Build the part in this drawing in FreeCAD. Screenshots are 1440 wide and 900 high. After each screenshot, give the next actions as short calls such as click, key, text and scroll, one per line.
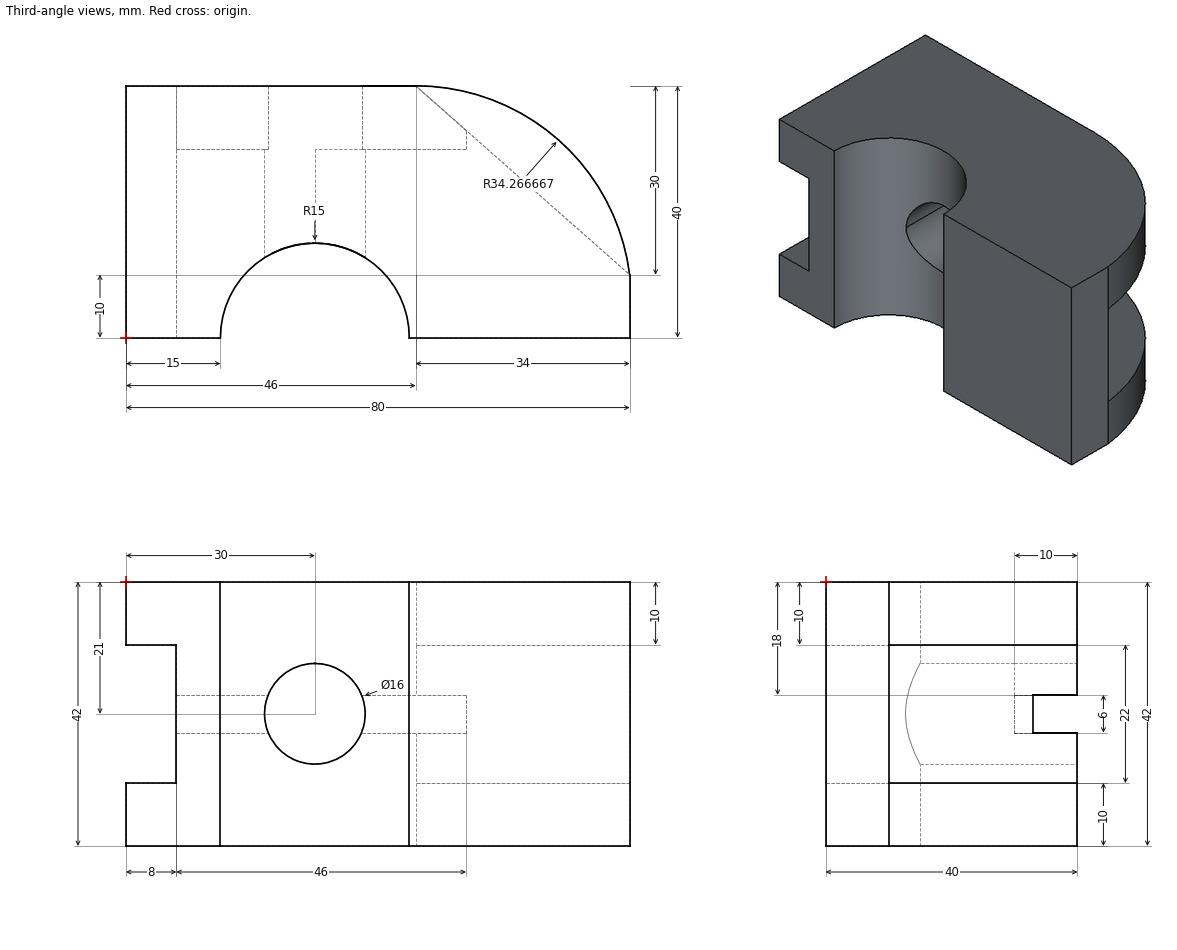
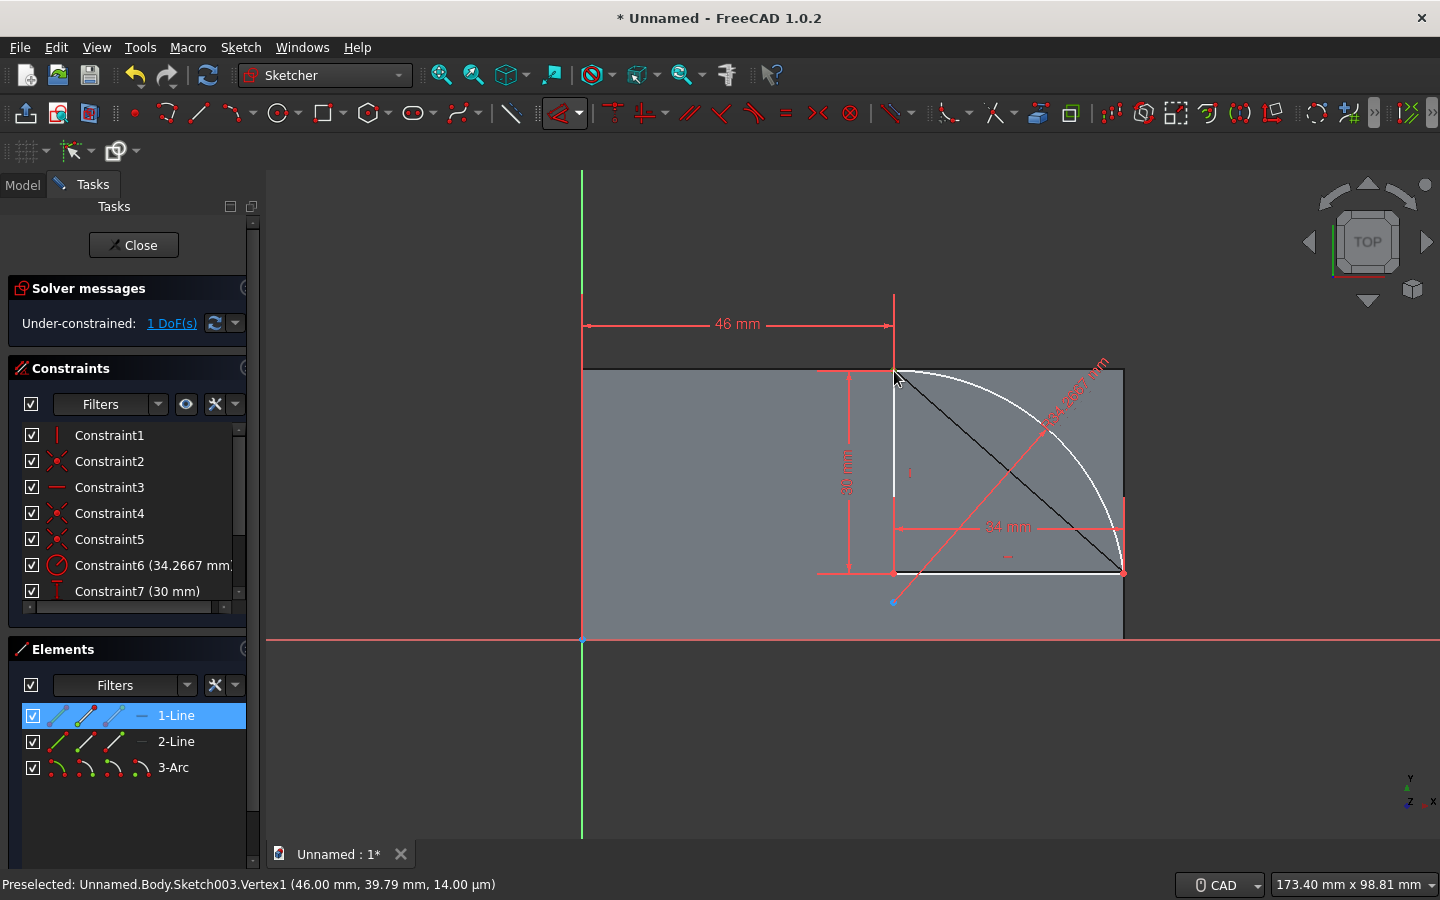
key(i)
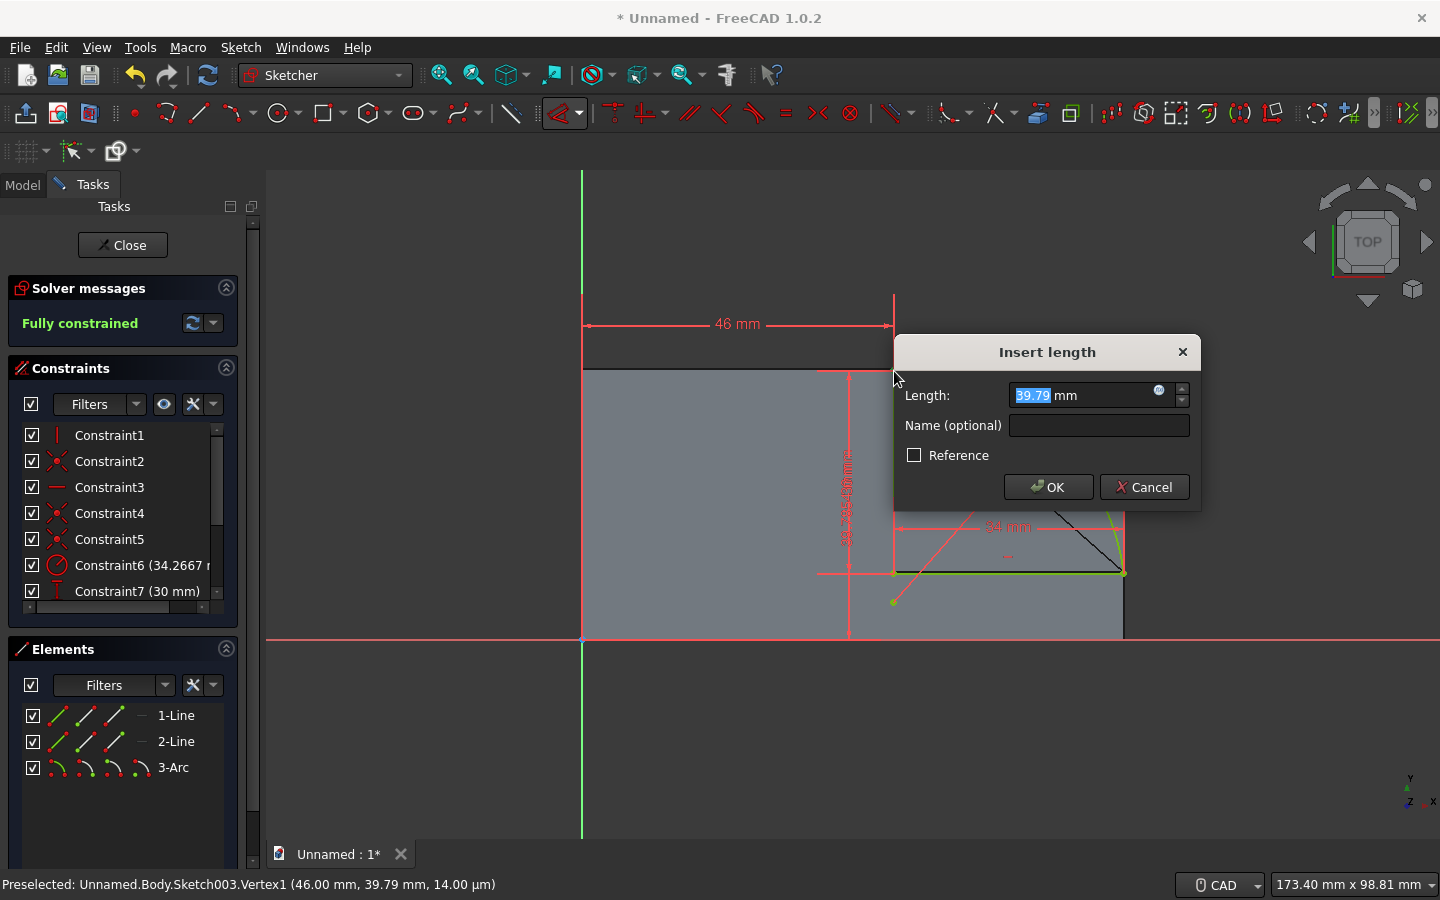
text(40)
key(Return)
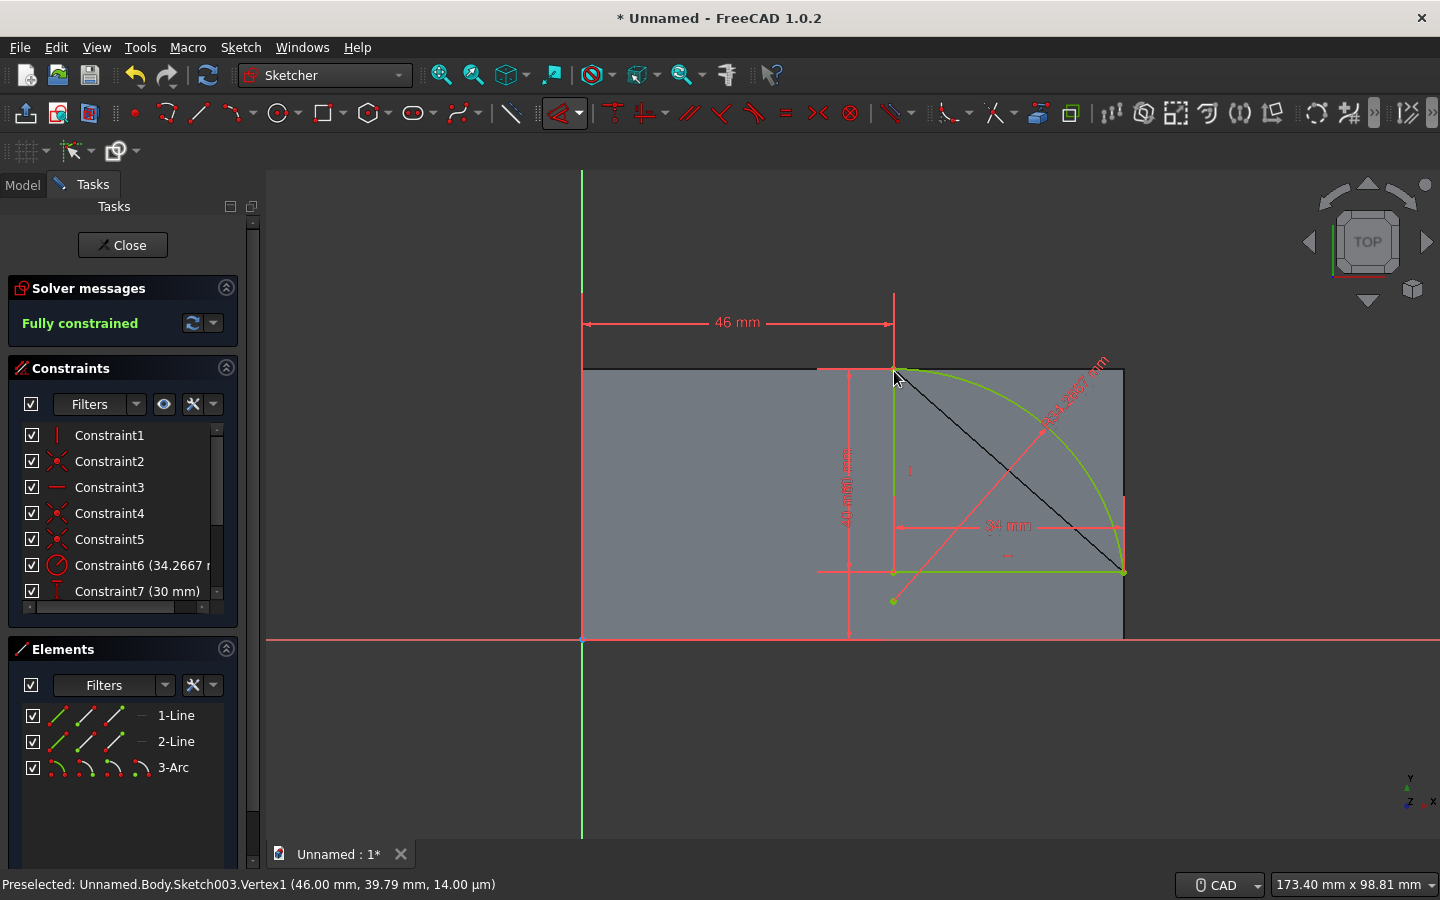
click(123, 245)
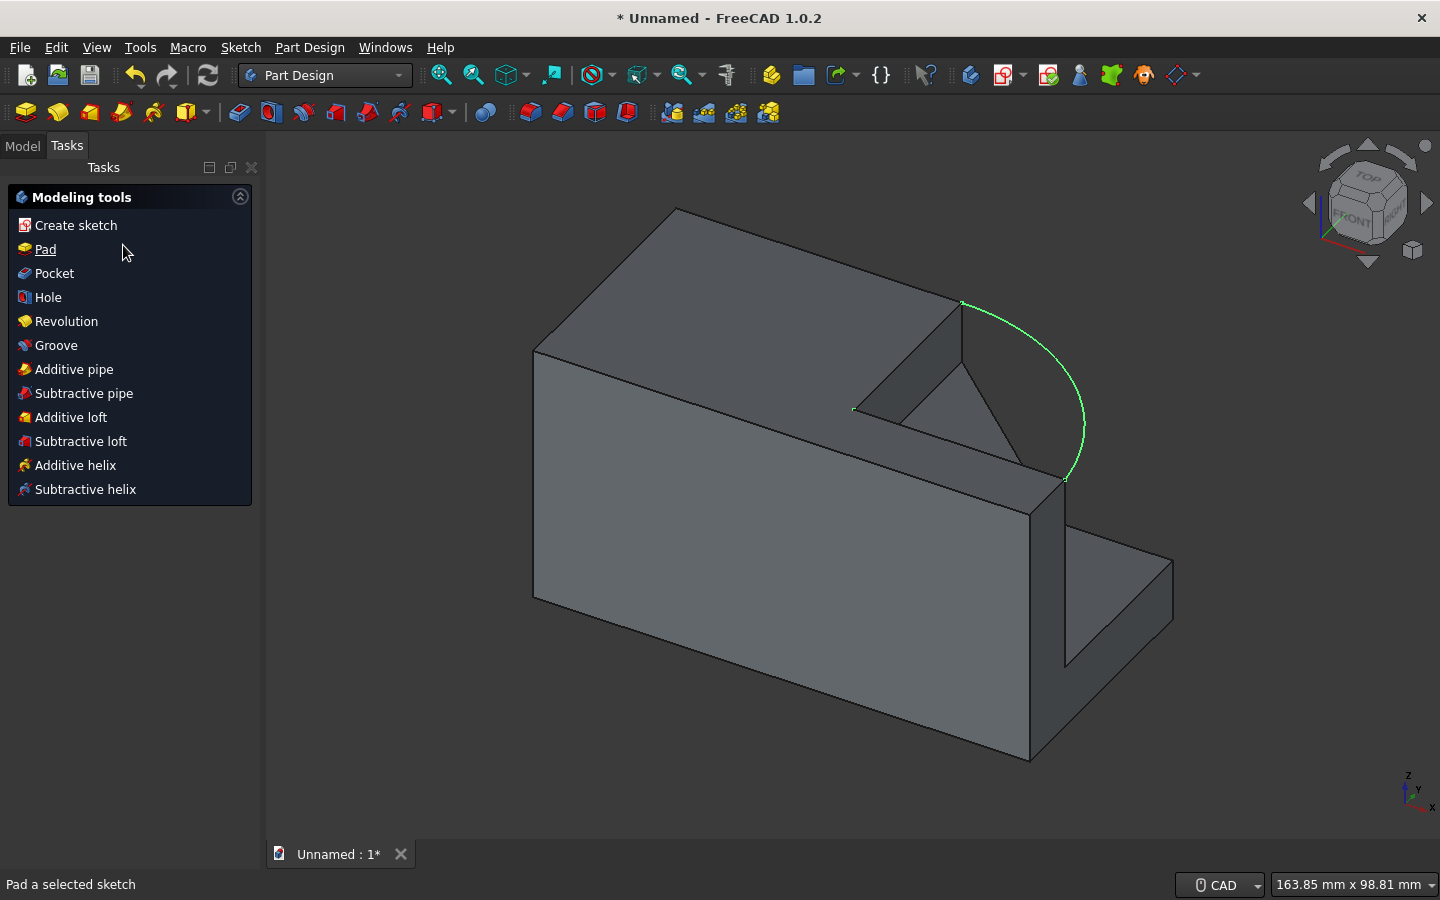
click(26, 112)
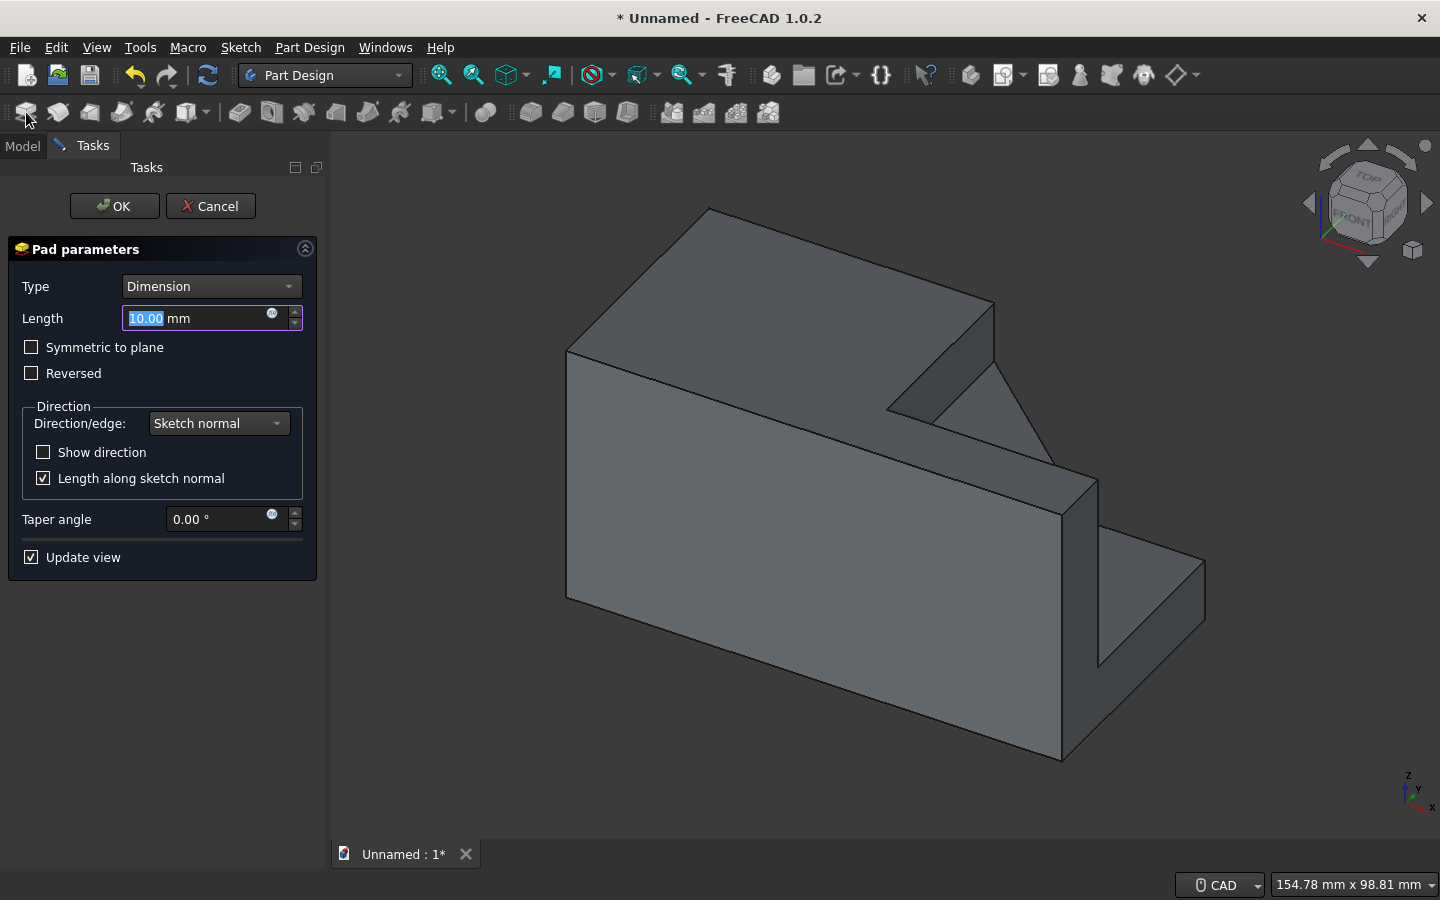
text(10)
key(Tab)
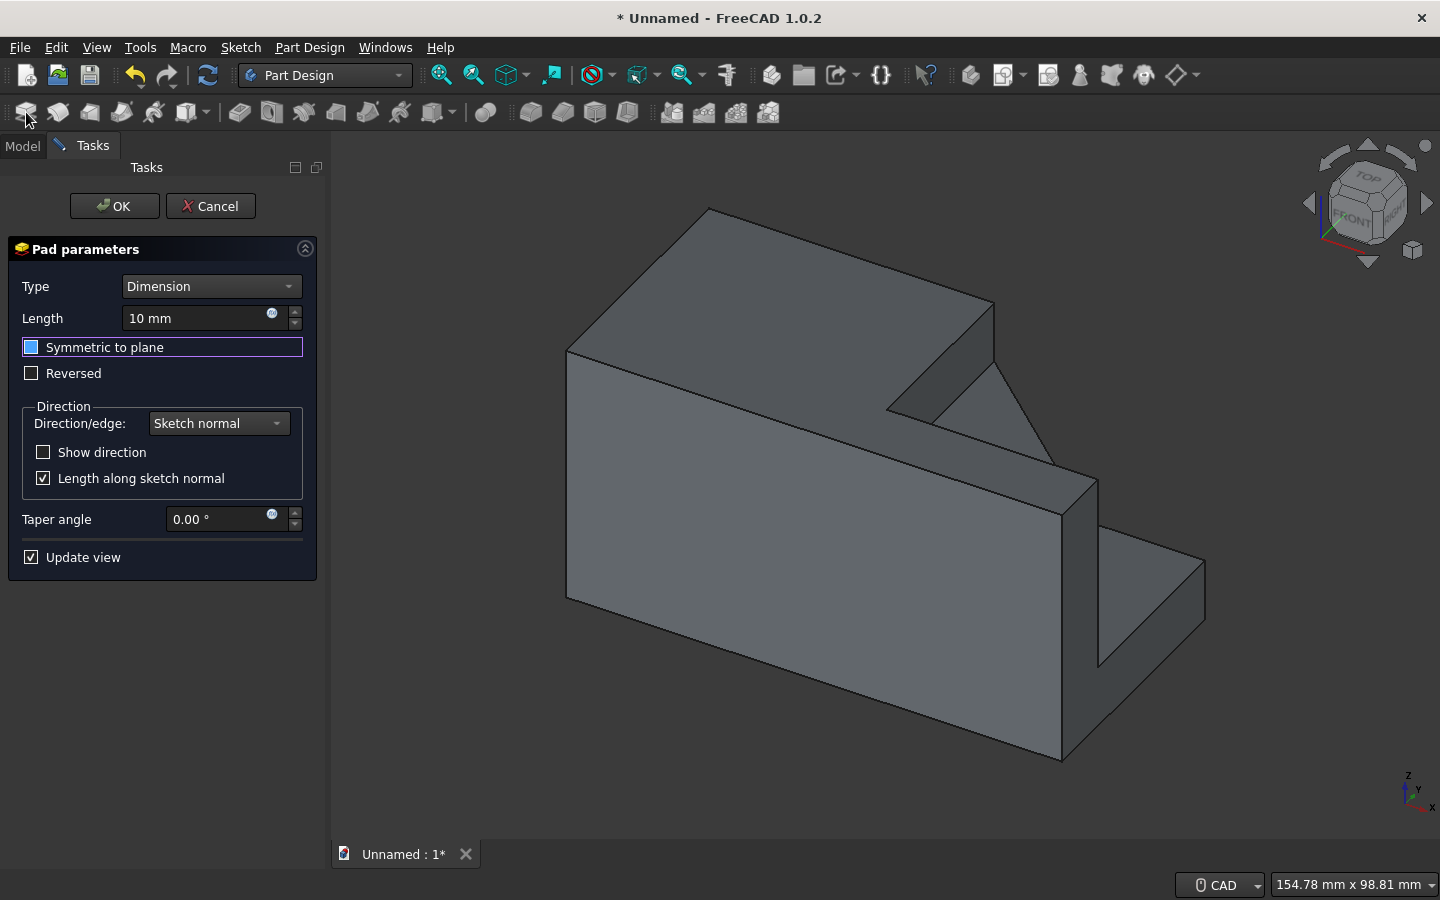
click(30, 373)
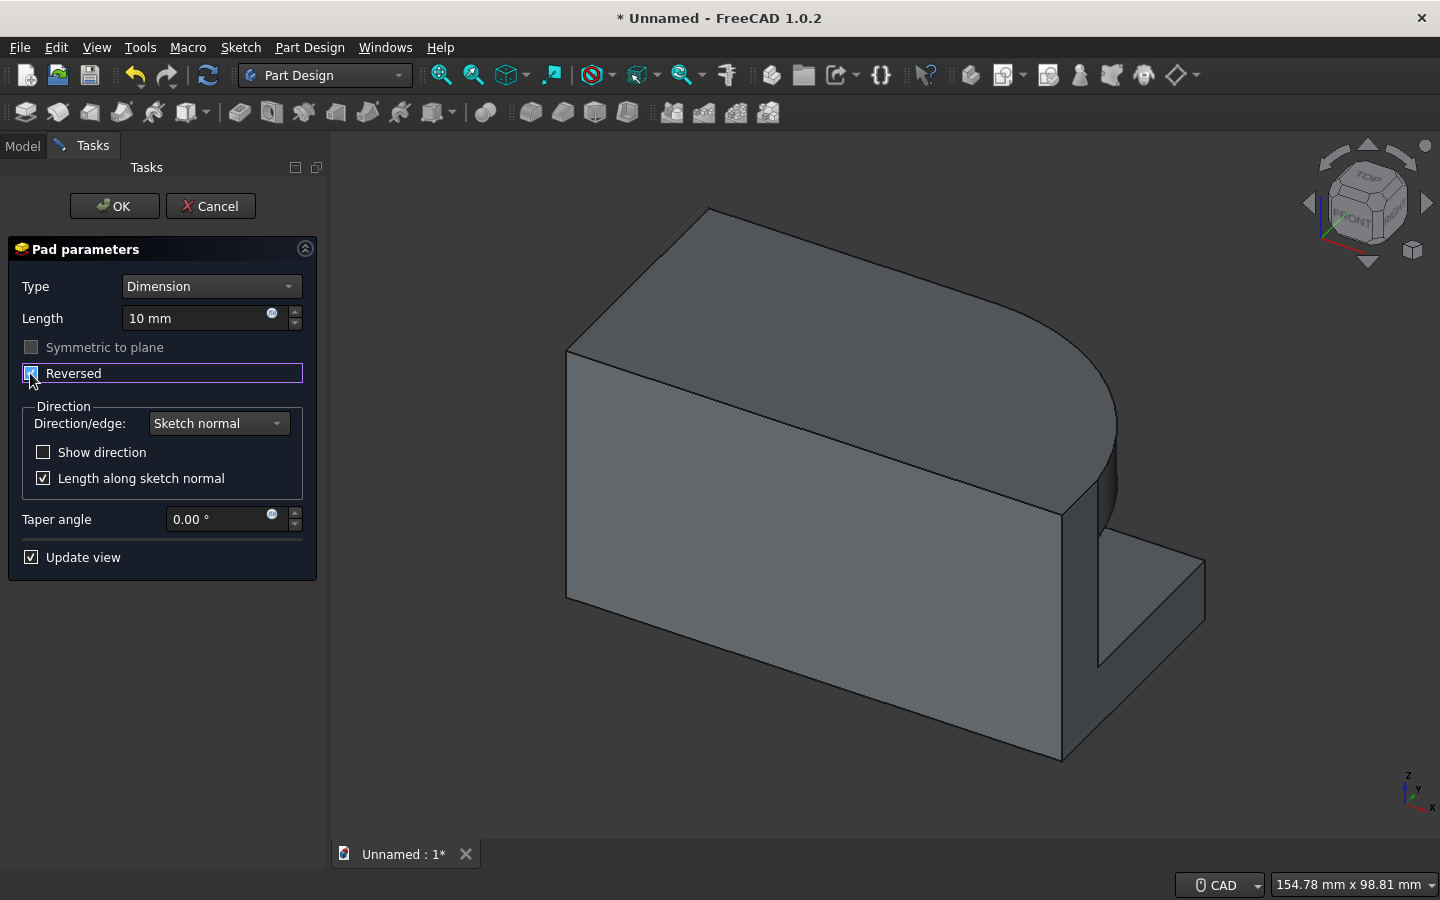
click(115, 206)